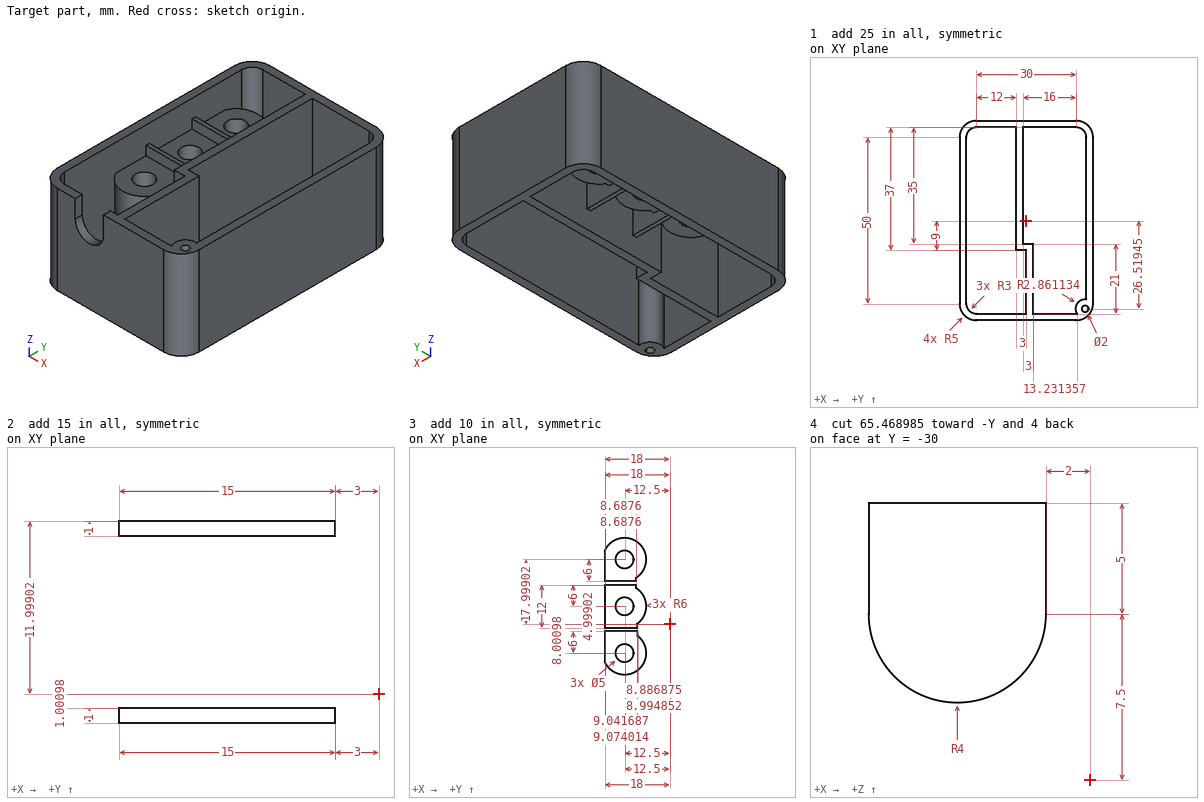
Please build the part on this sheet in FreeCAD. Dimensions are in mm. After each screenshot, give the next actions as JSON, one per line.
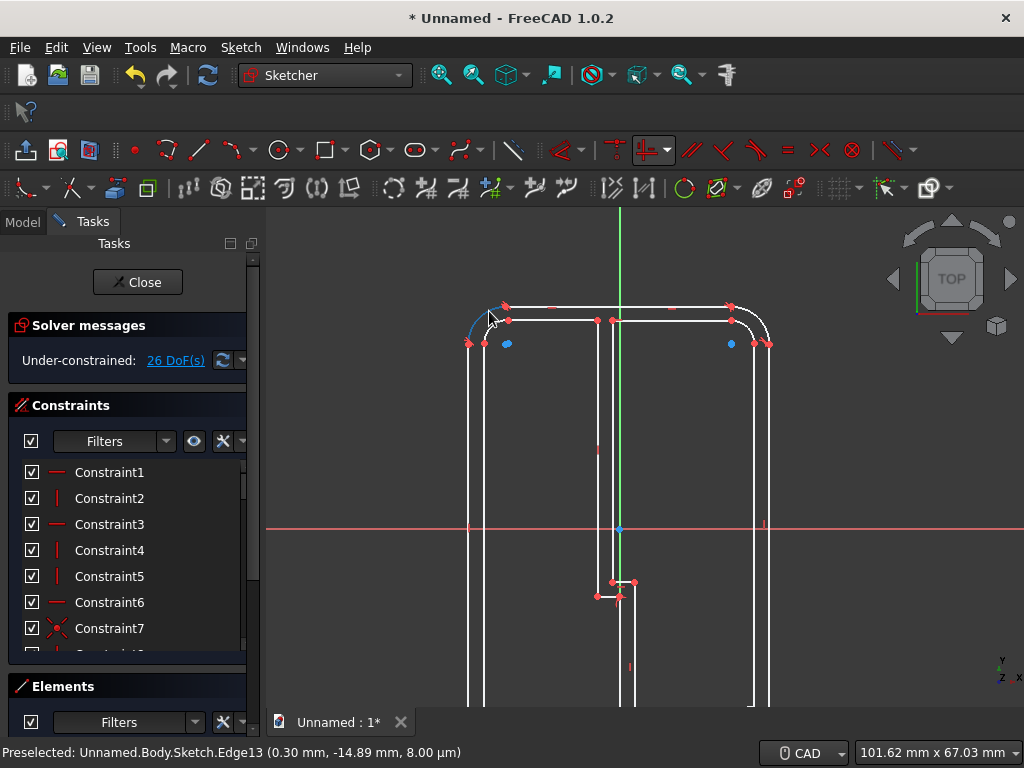
{"action": "left_click", "coordinate": [489, 311]}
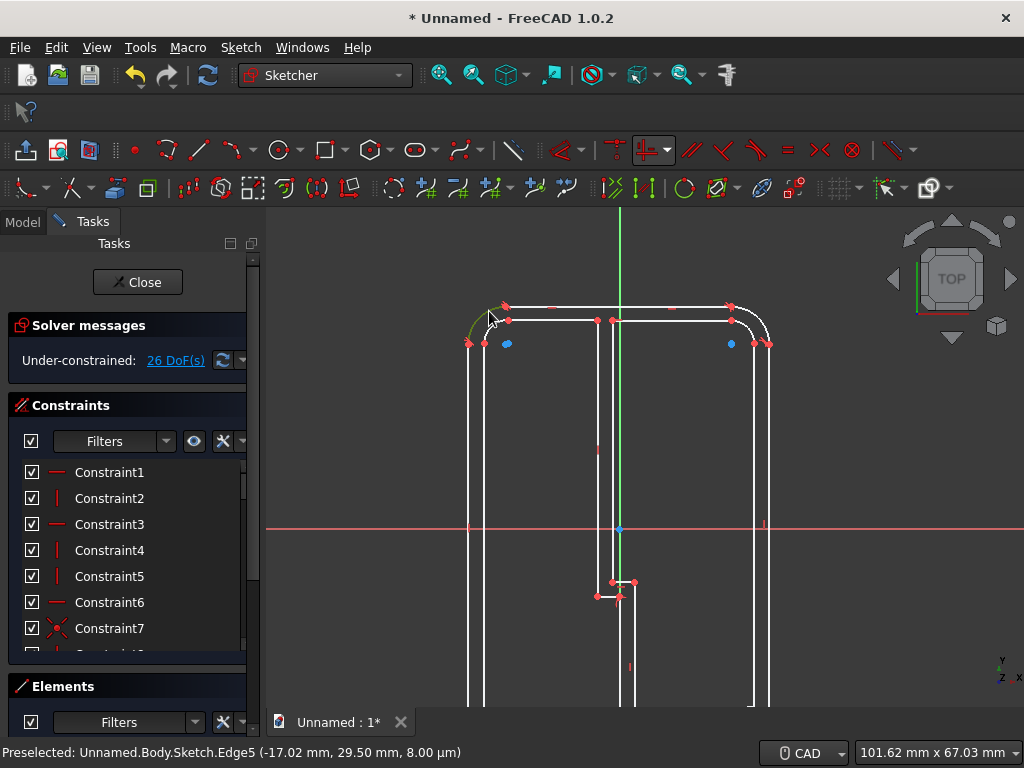
{"action": "scroll", "coordinate": [497, 323], "scroll_direction": "up", "scroll_amount": 2}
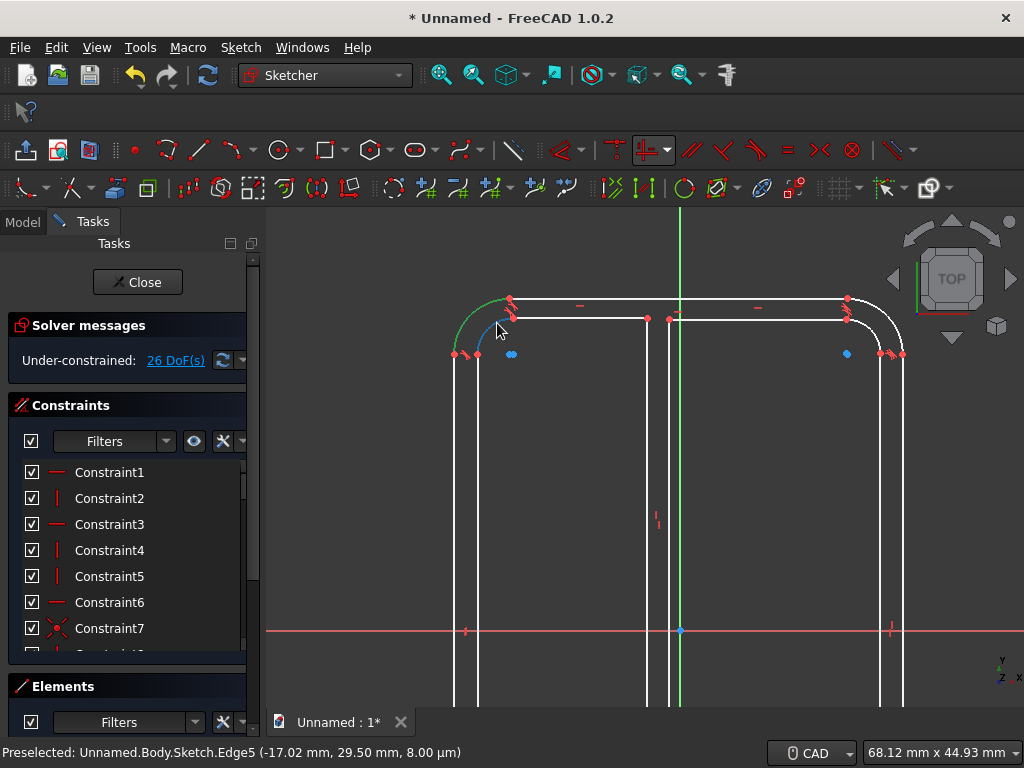
{"action": "left_click", "coordinate": [497, 322]}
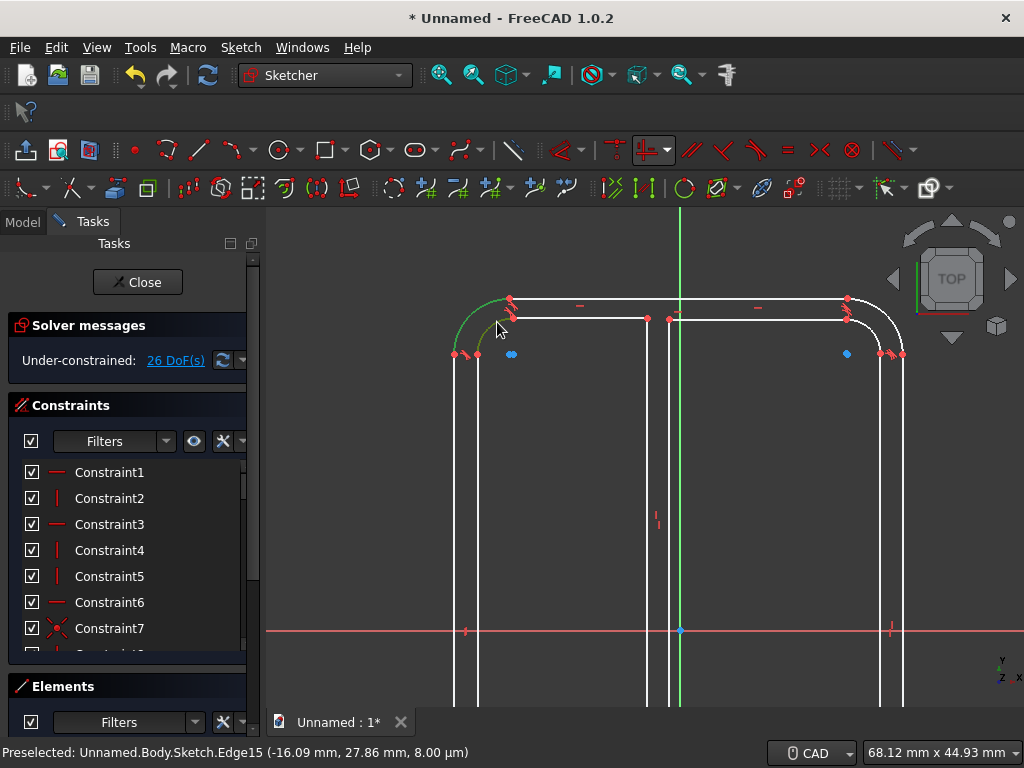
{"action": "left_click", "coordinate": [616, 150]}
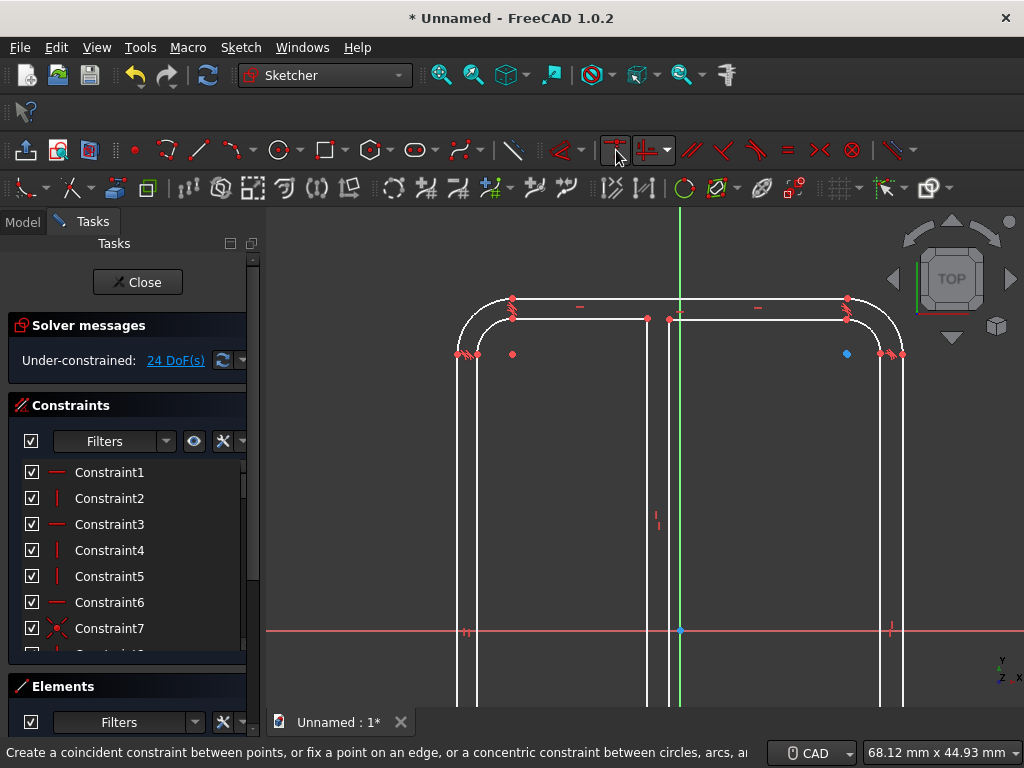
{"action": "scroll", "coordinate": [492, 315], "scroll_direction": "down", "scroll_amount": 4}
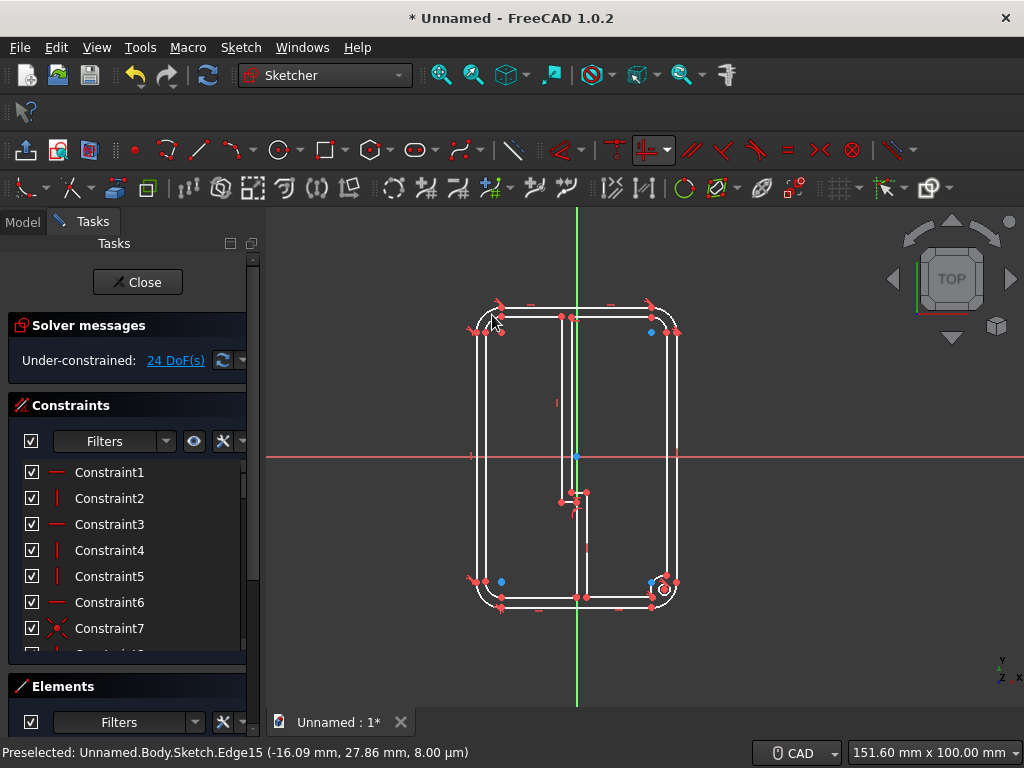
{"action": "scroll", "coordinate": [479, 594], "scroll_direction": "up", "scroll_amount": 2}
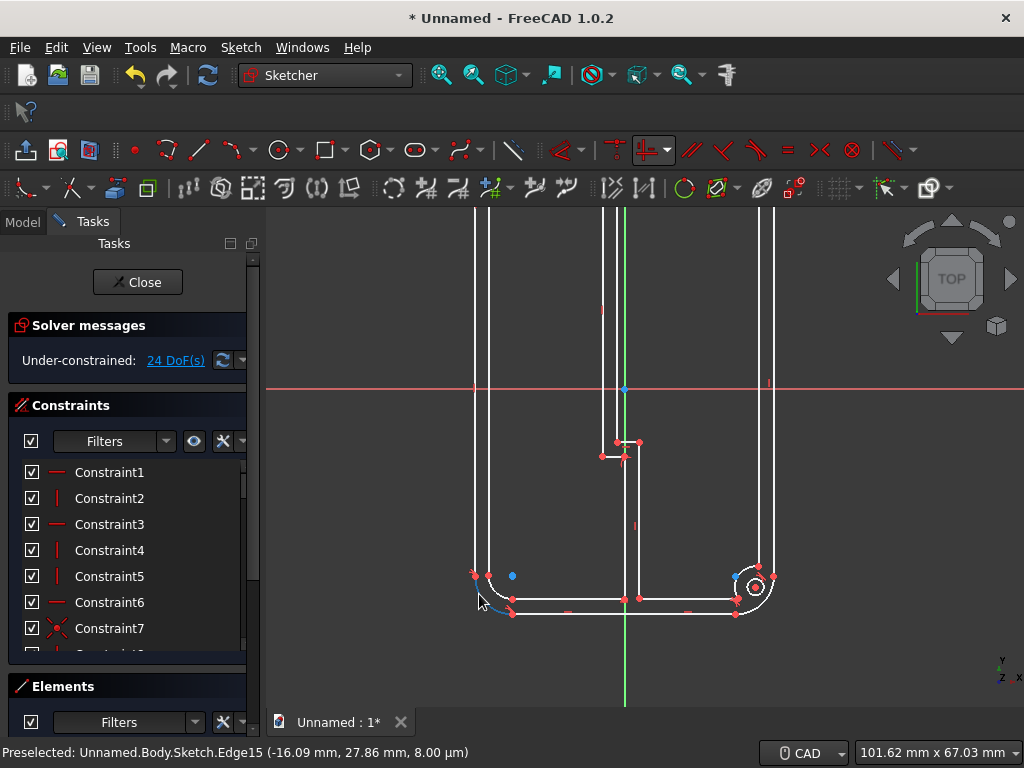
{"action": "left_click", "coordinate": [479, 594]}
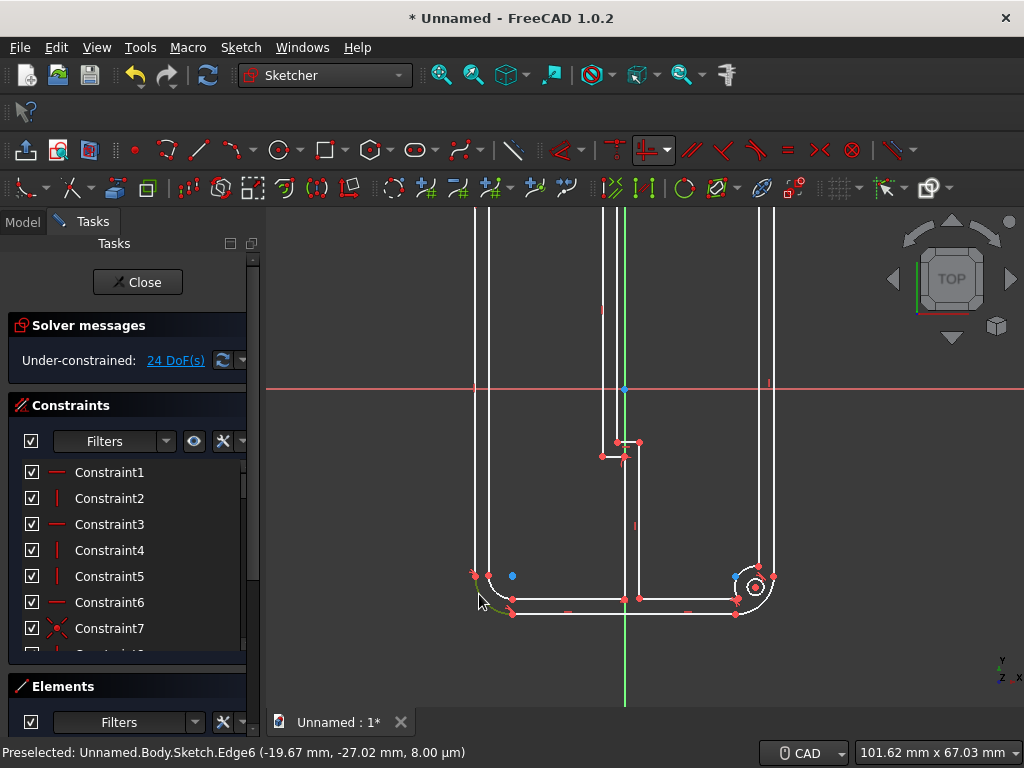
{"action": "scroll", "coordinate": [491, 586], "scroll_direction": "up", "scroll_amount": 2}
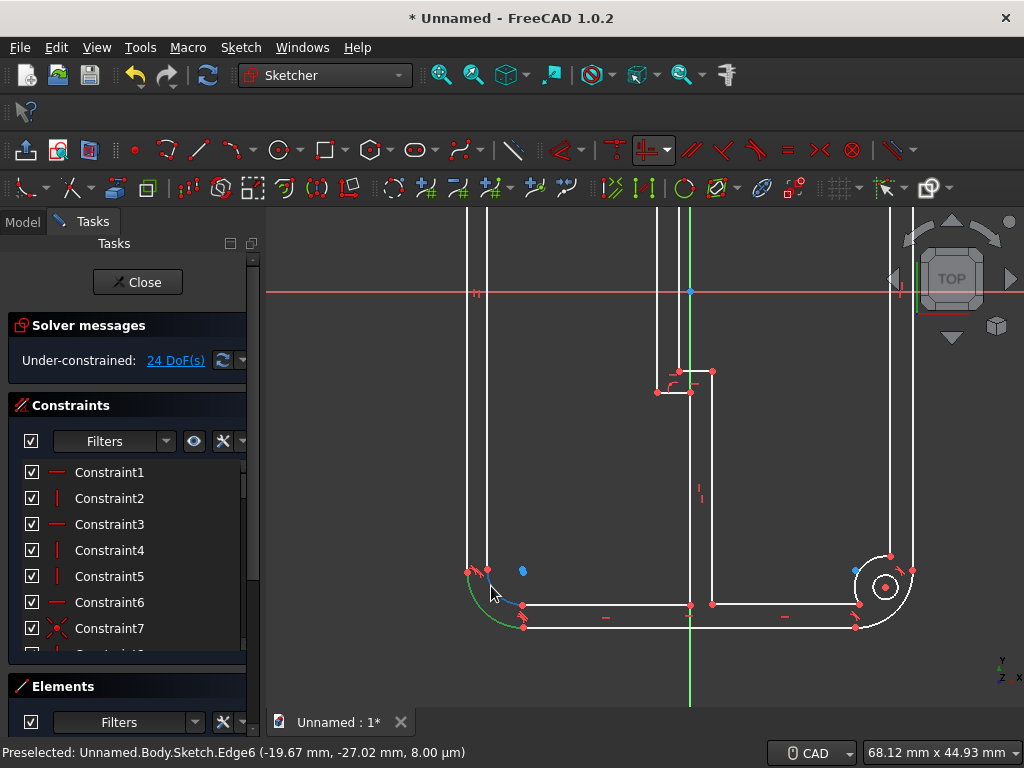
{"action": "left_click", "coordinate": [491, 586]}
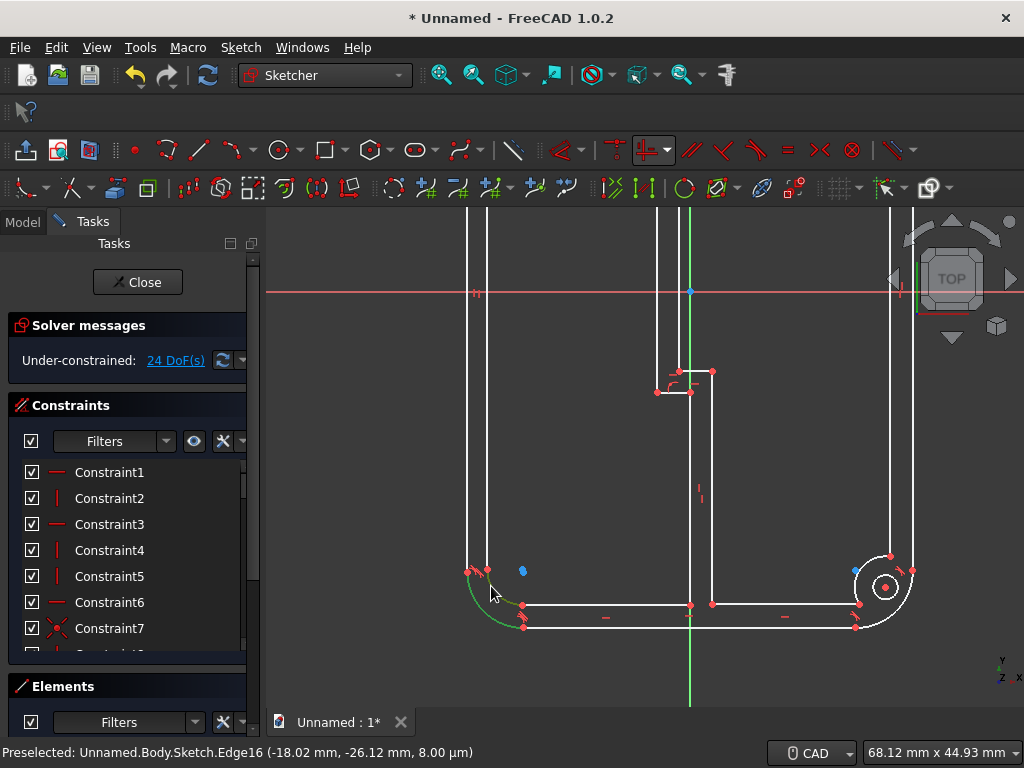
{"action": "left_click", "coordinate": [616, 150]}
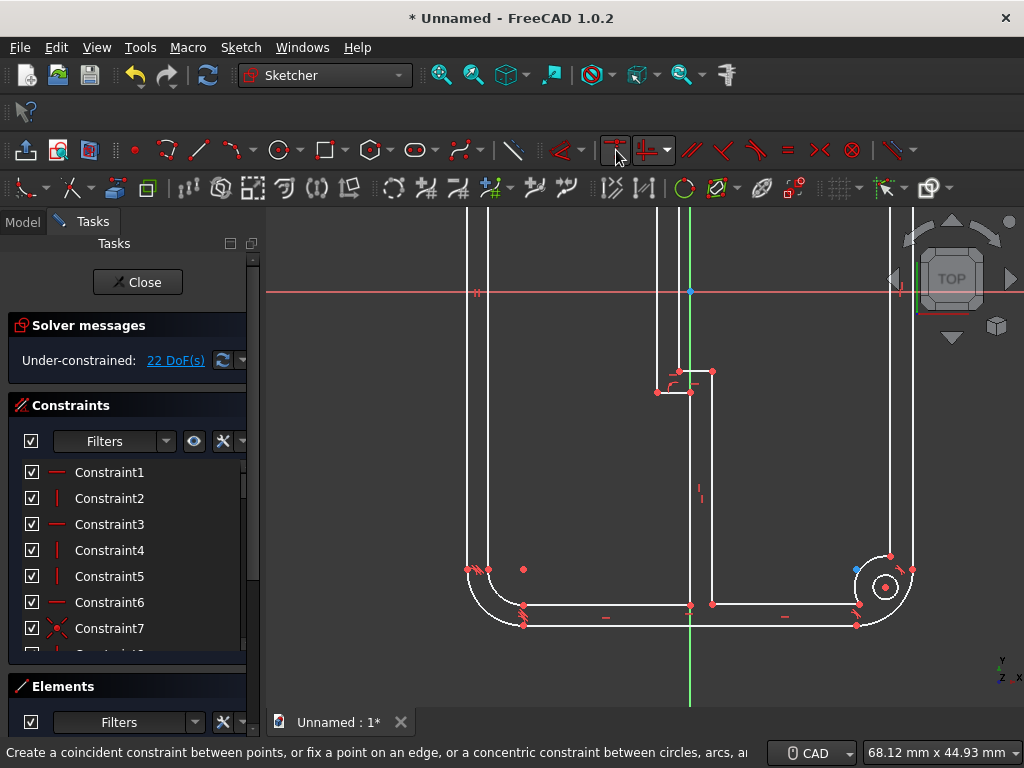
{"action": "scroll", "coordinate": [484, 592], "scroll_direction": "down", "scroll_amount": 4}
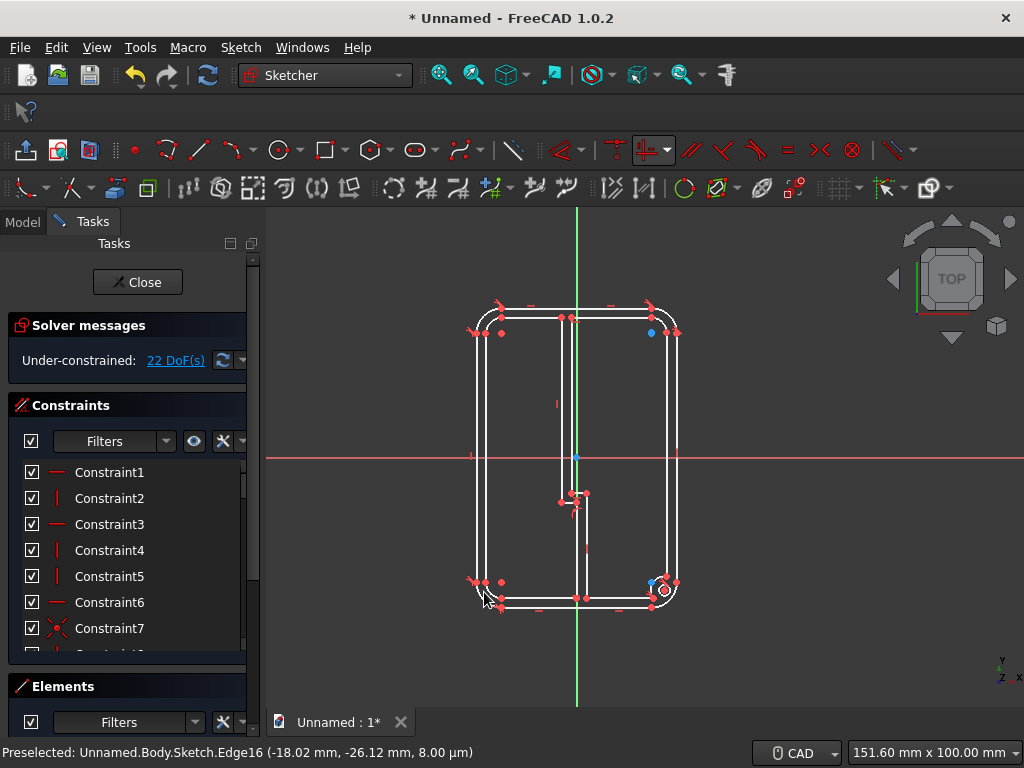
{"action": "scroll", "coordinate": [674, 322], "scroll_direction": "up", "scroll_amount": 2}